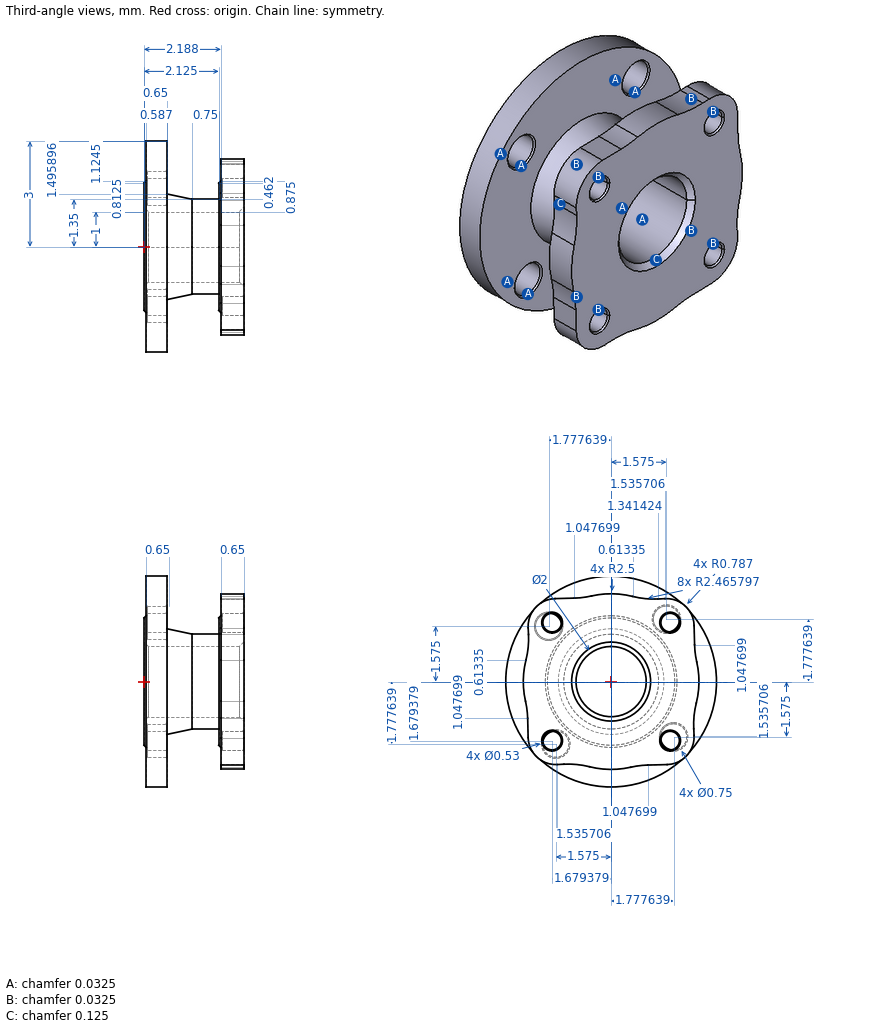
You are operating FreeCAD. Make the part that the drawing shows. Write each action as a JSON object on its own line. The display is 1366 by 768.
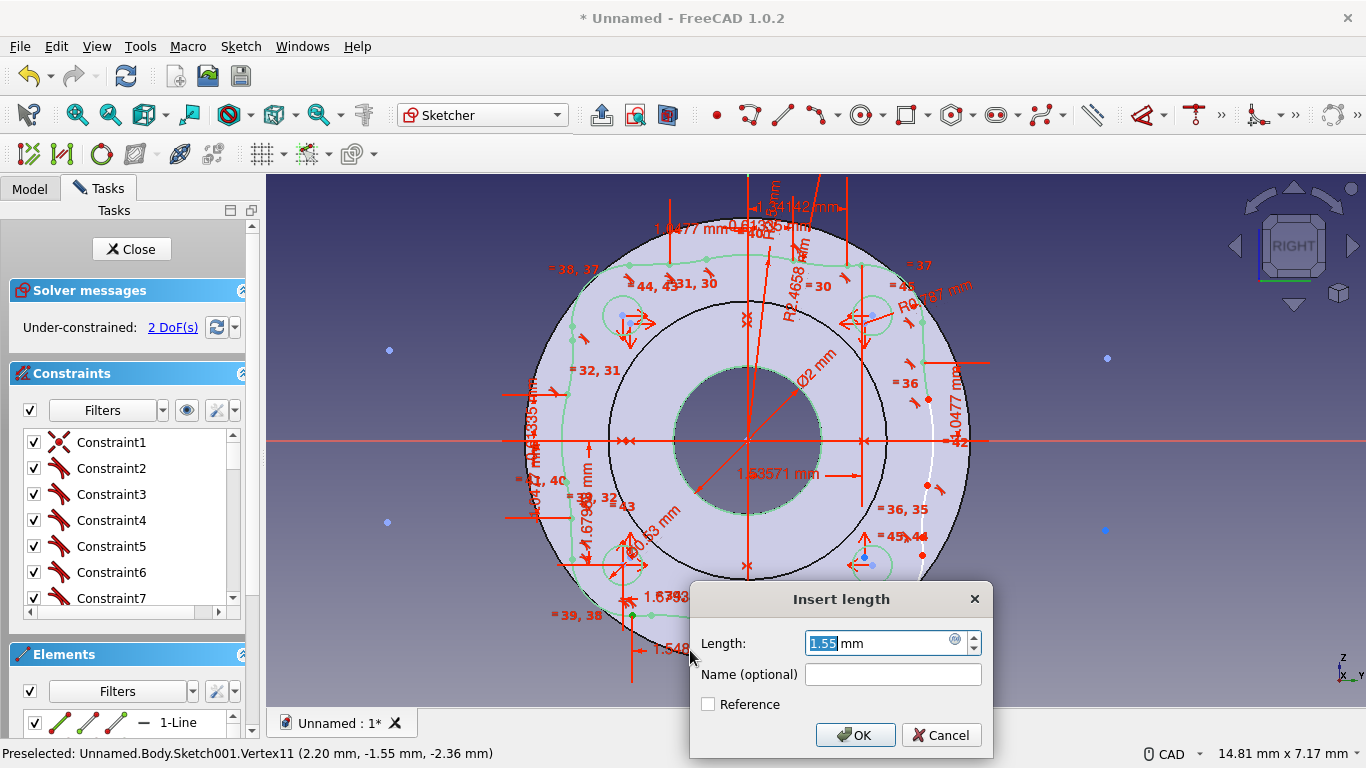
{"action": "type", "text": "1.535706"}
{"action": "key", "text": "Return"}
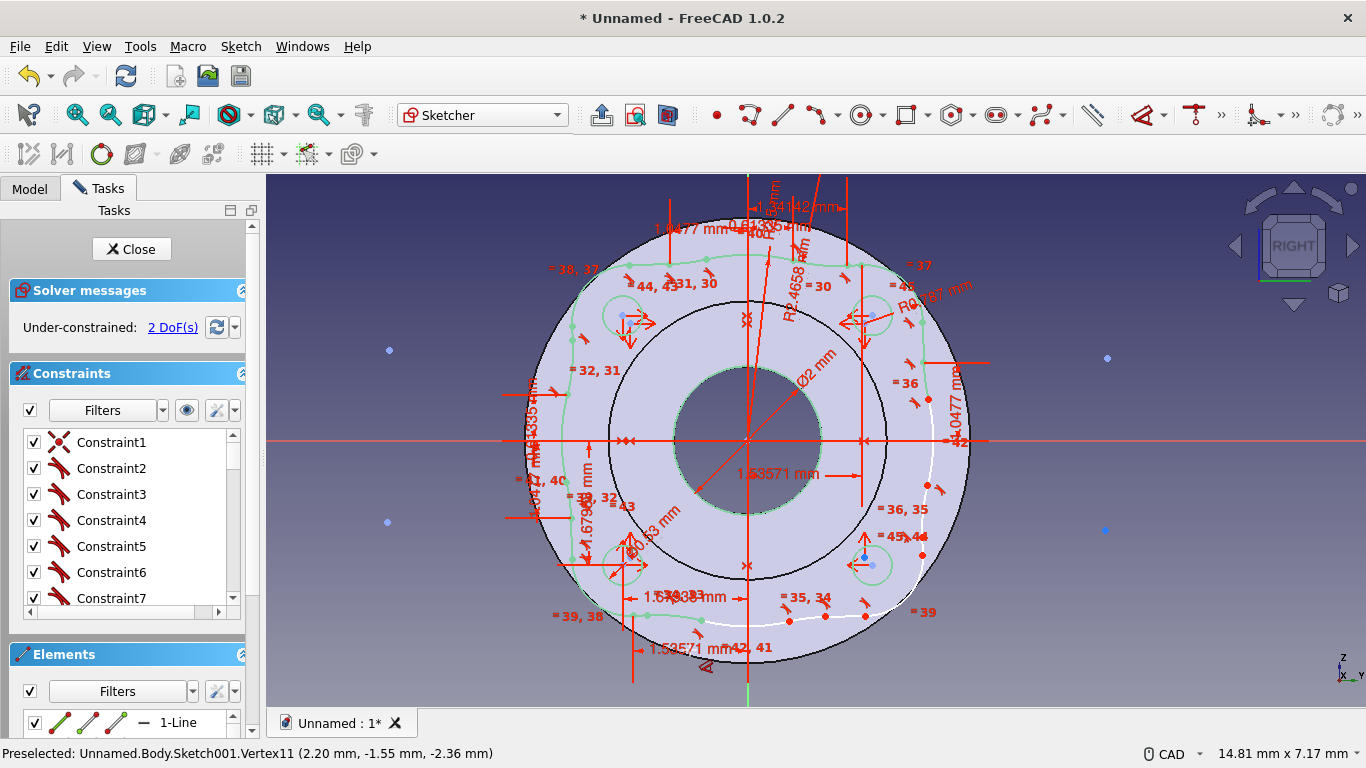
{"action": "left_click", "coordinate": [826, 617]}
{"action": "left_click", "coordinate": [787, 651]}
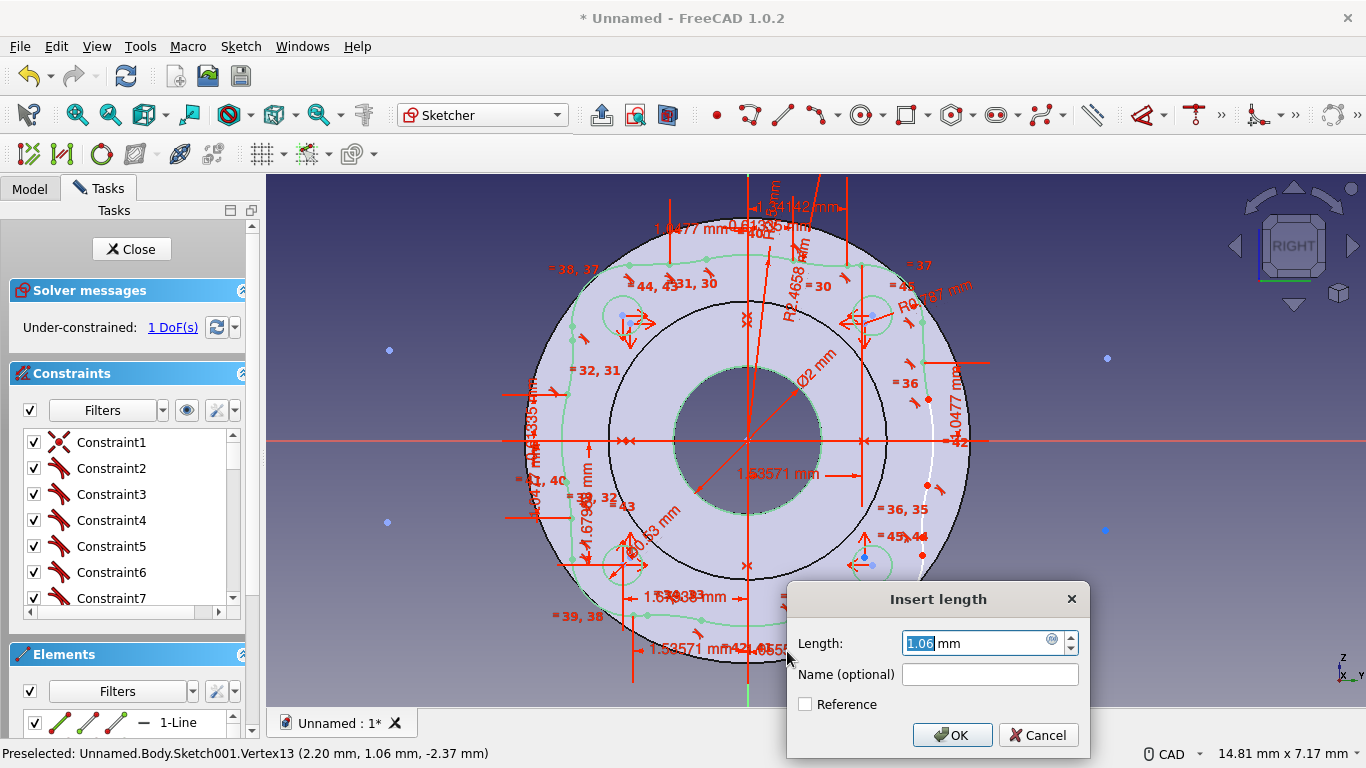
{"action": "type", "text": "1.047699"}
{"action": "key", "text": "Return"}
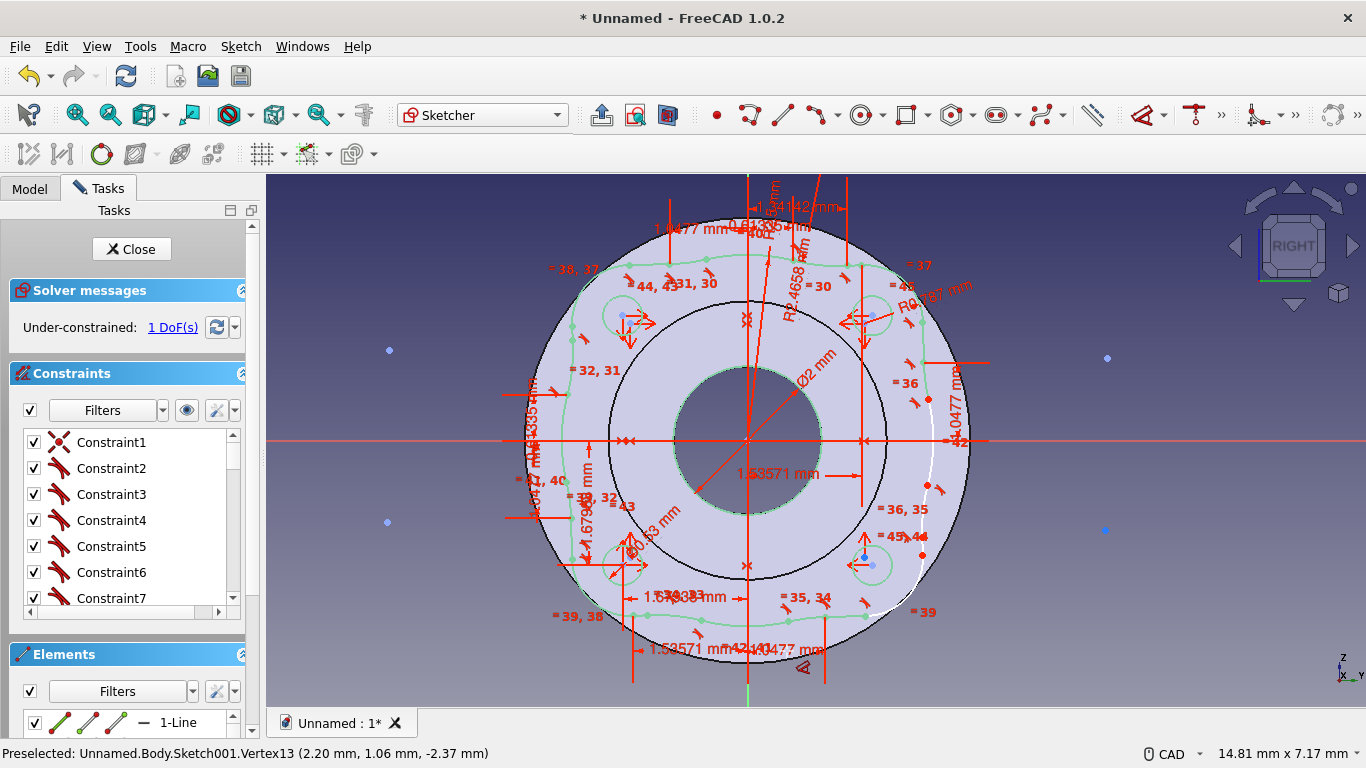
{"action": "left_click", "coordinate": [923, 555]}
{"action": "left_click", "coordinate": [957, 498]}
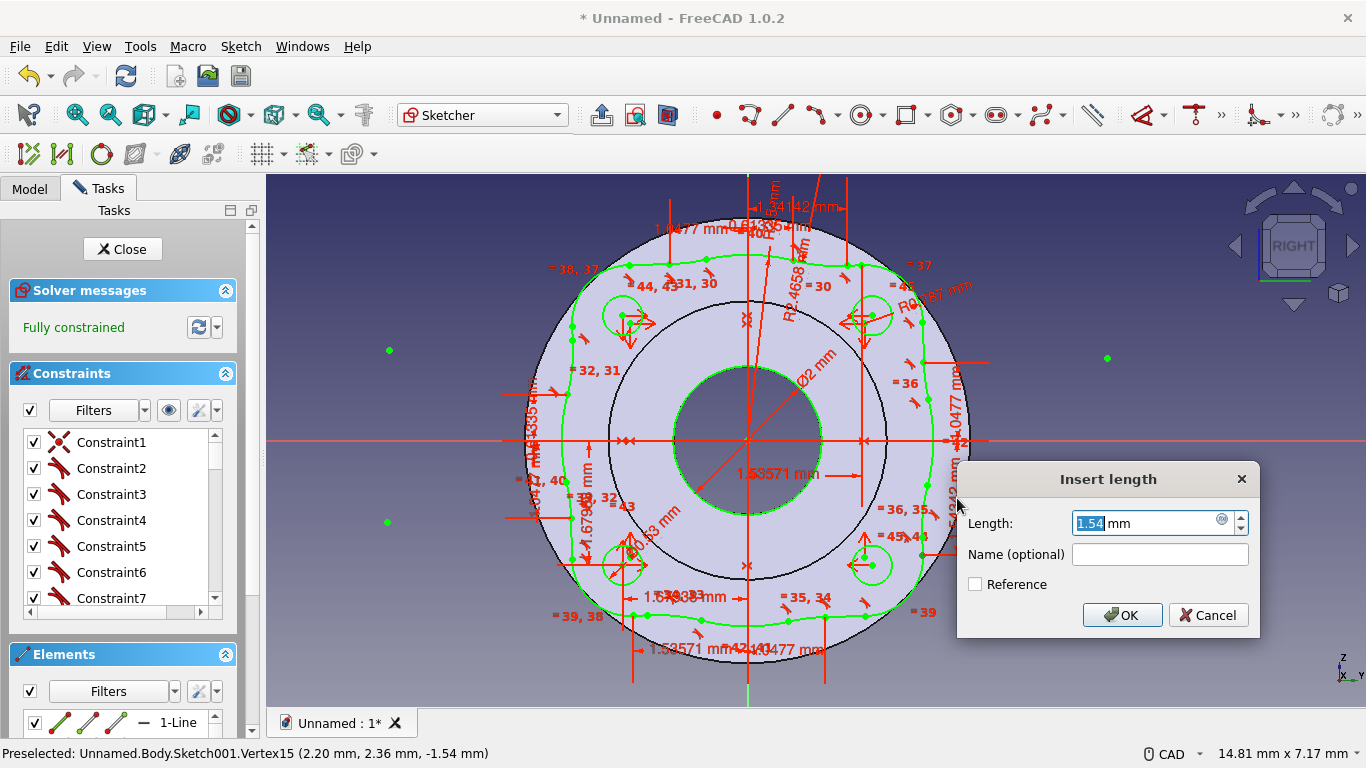
{"action": "type", "text": "1.535706"}
{"action": "key", "text": "Return"}
{"action": "key", "text": "Escape"}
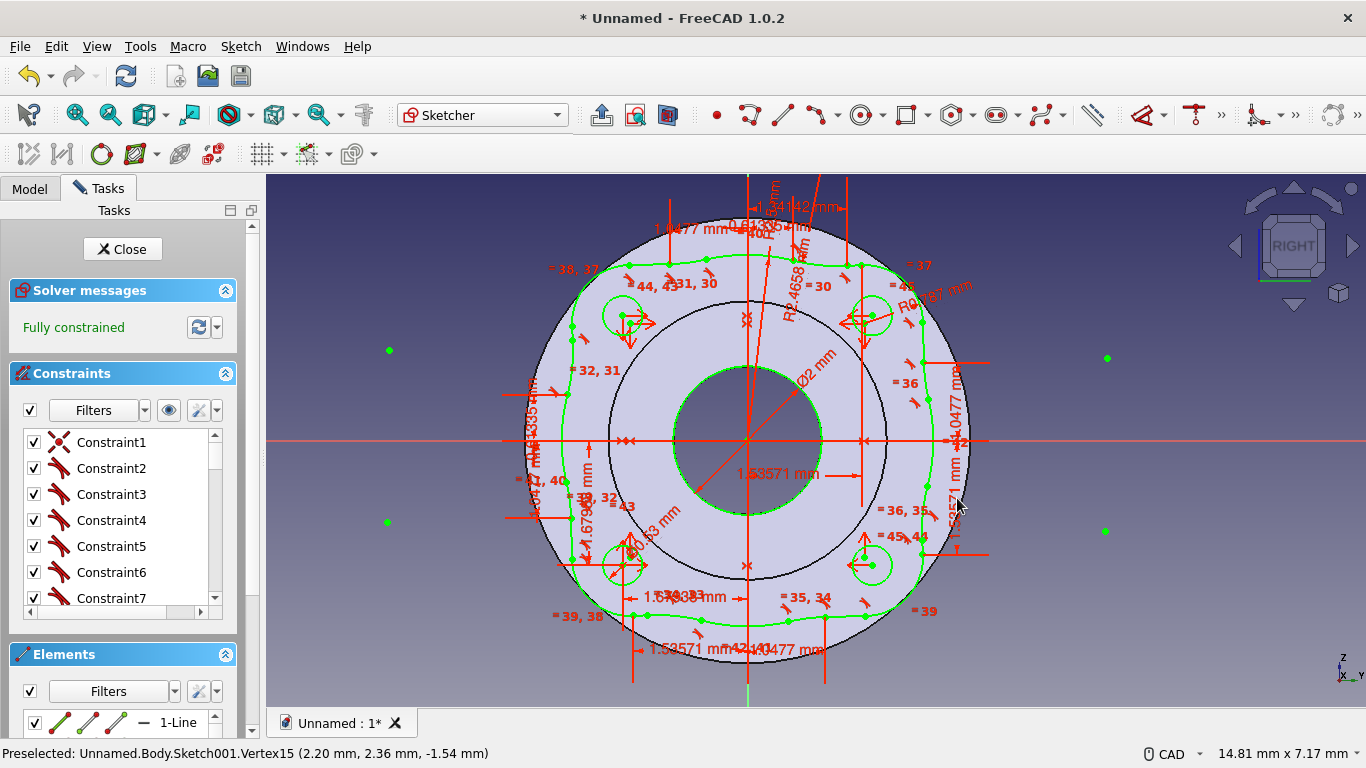
{"action": "left_click", "coordinate": [123, 249]}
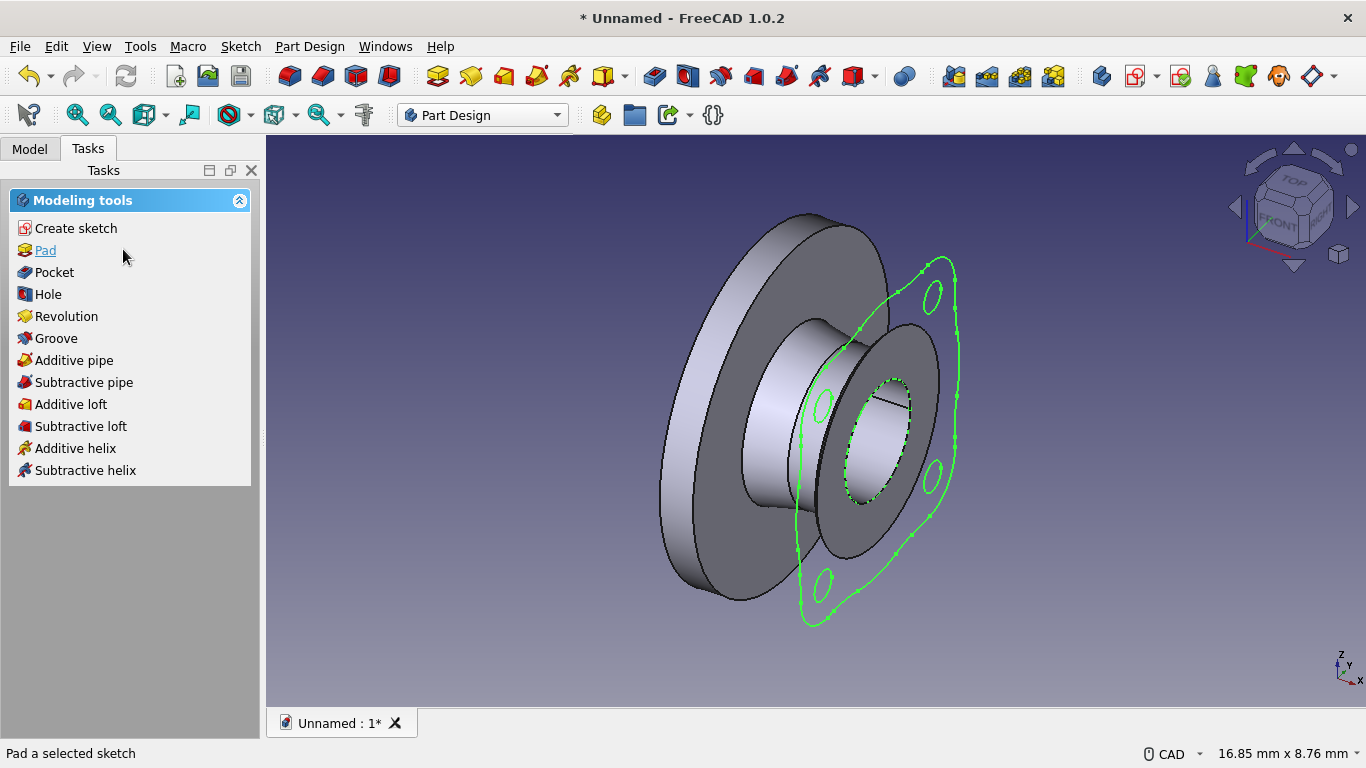
{"action": "left_click", "coordinate": [438, 76]}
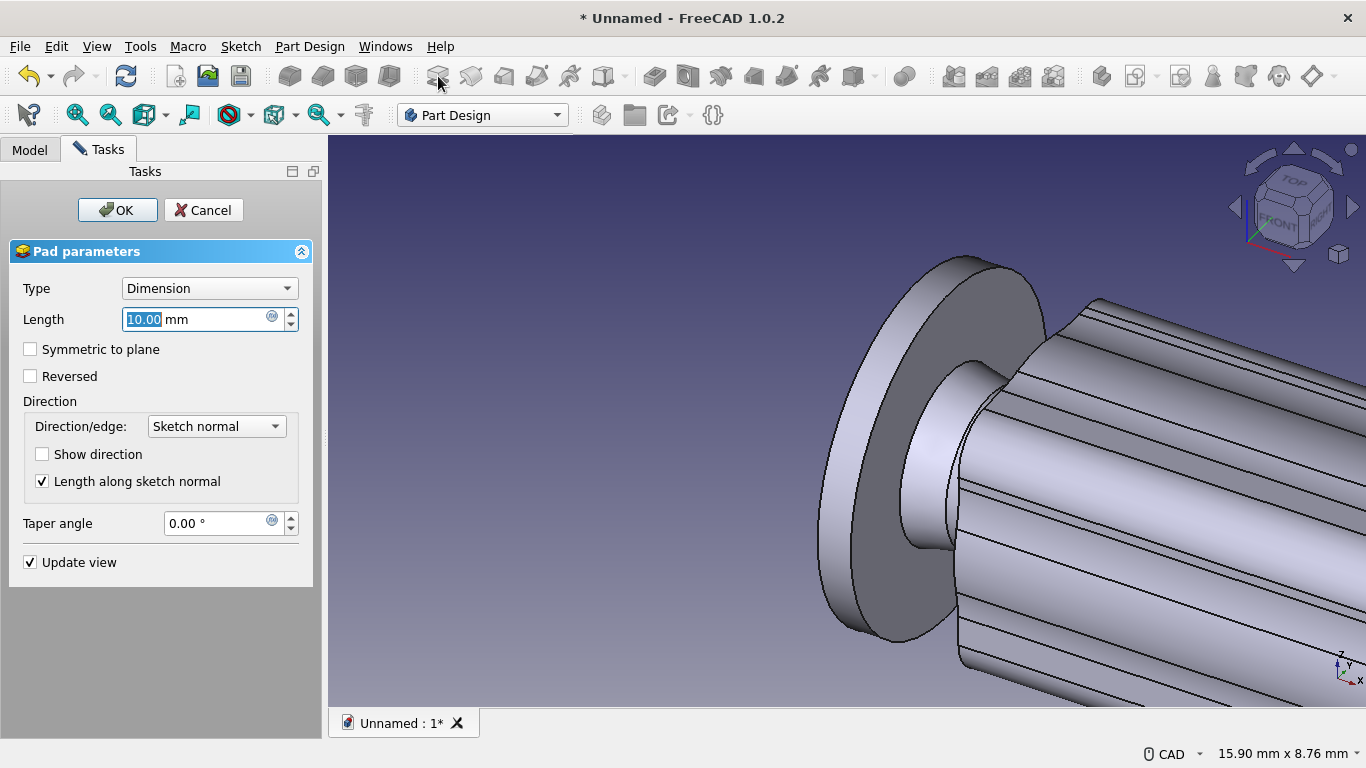
{"action": "type", "text": "0.65"}
{"action": "key", "text": "Tab"}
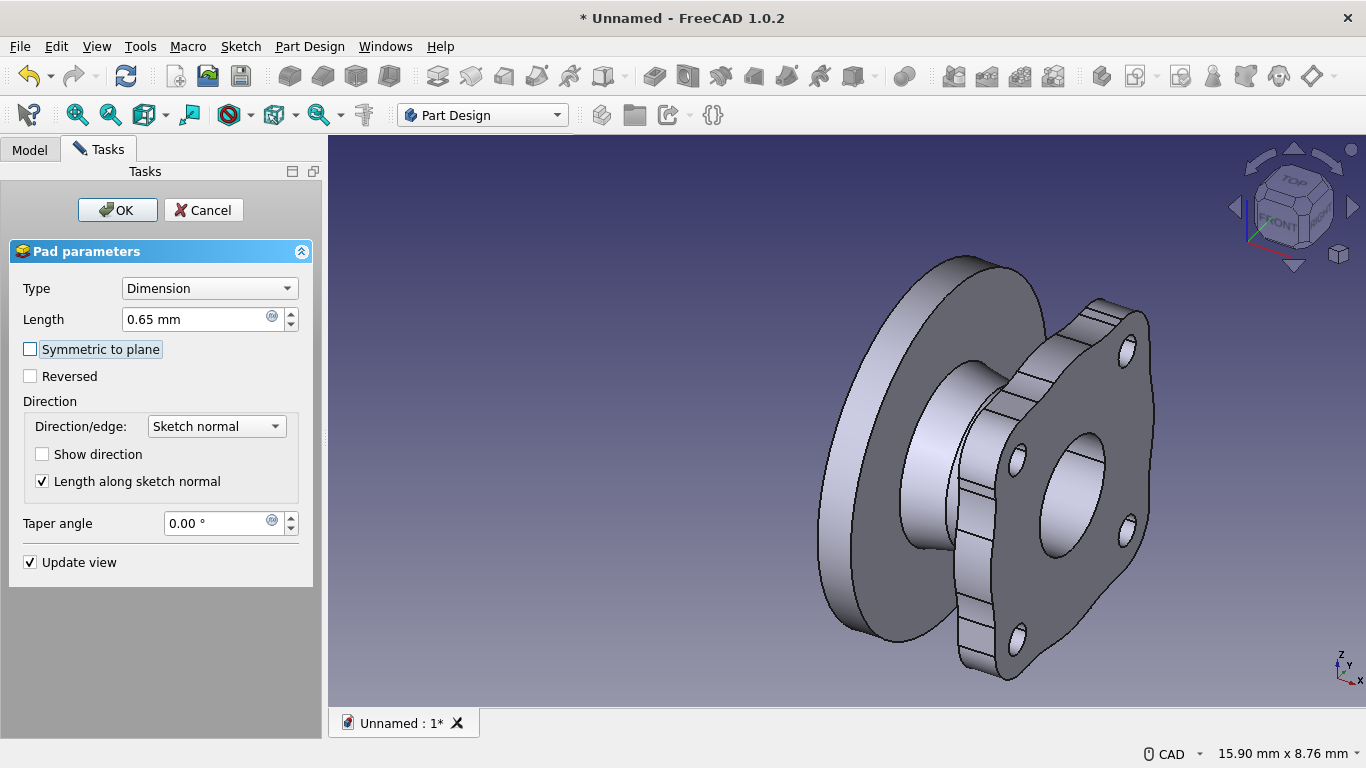
{"action": "left_click", "coordinate": [118, 210]}